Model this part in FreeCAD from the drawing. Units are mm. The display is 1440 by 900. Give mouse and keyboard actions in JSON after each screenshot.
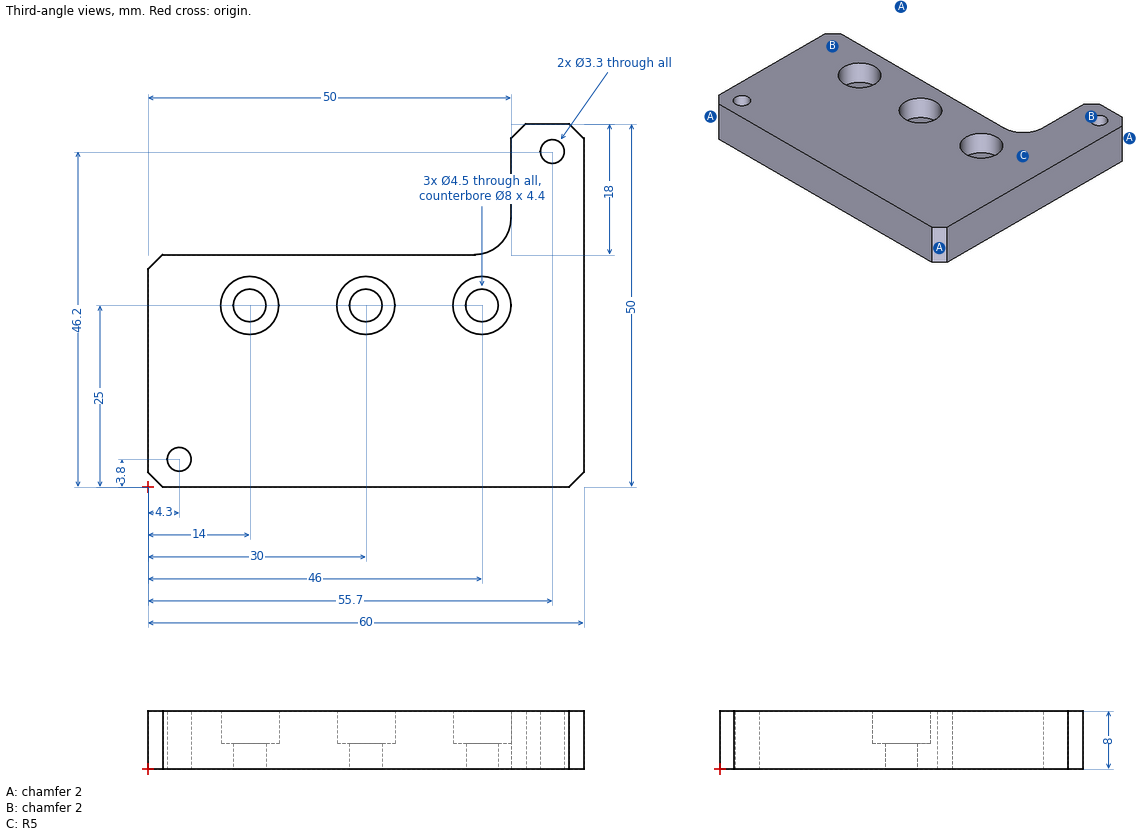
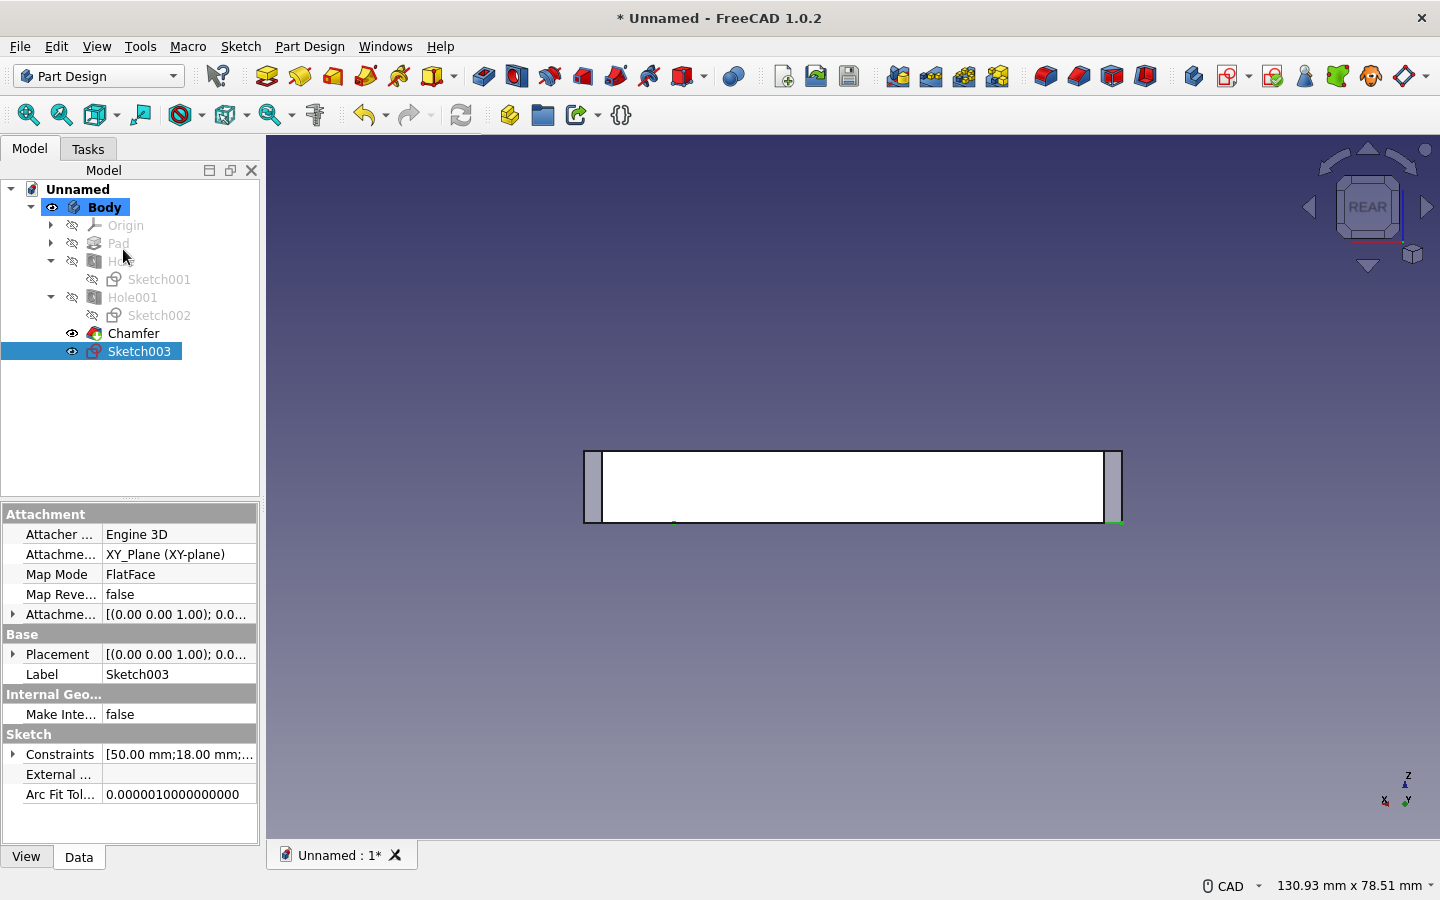
{"action": "left_click", "coordinate": [484, 76]}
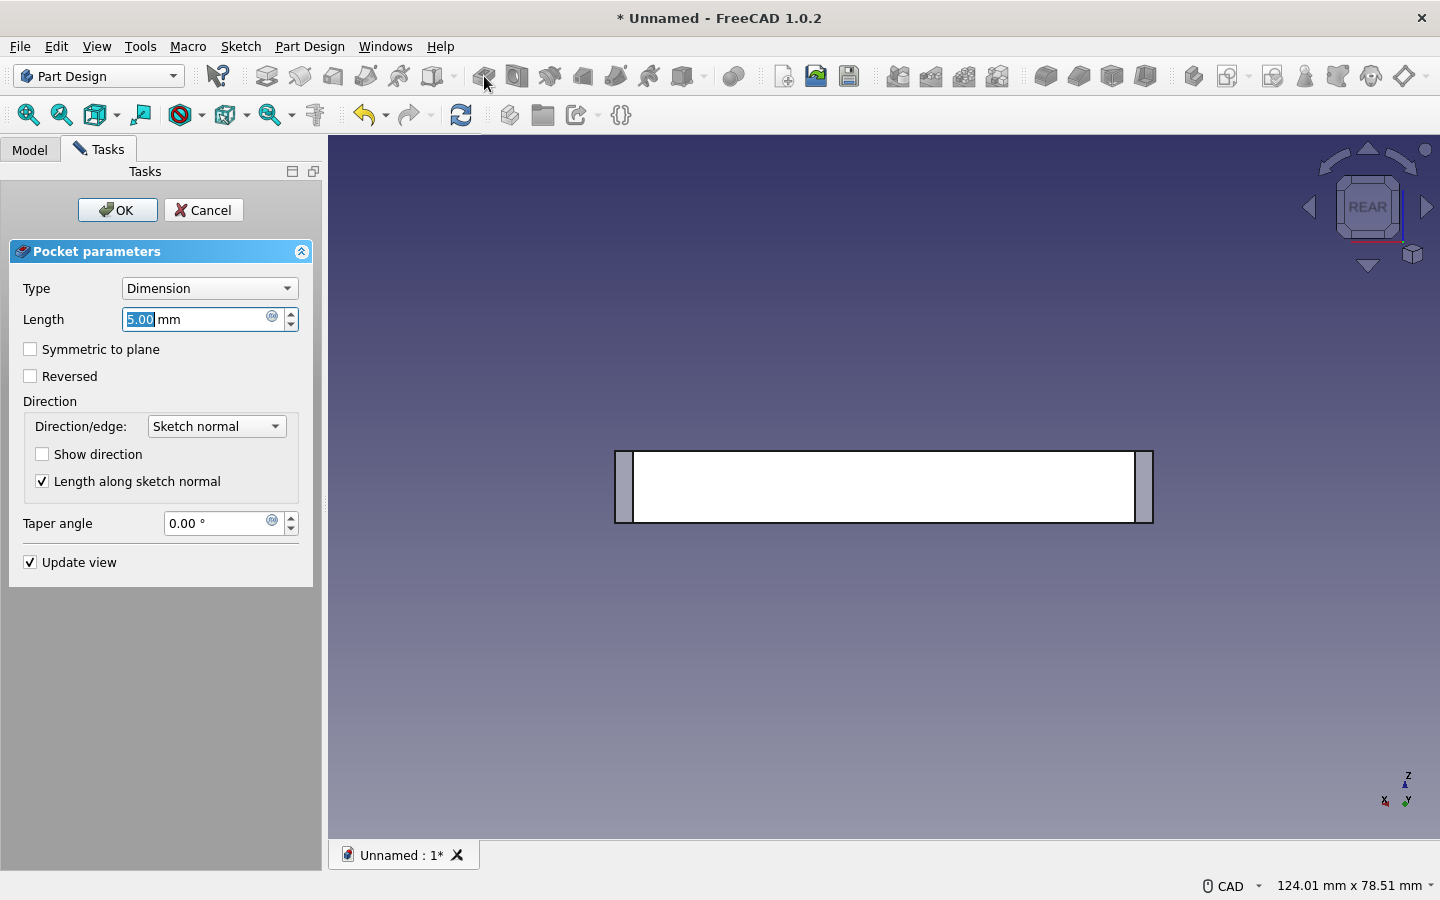
{"action": "left_click", "coordinate": [210, 288]}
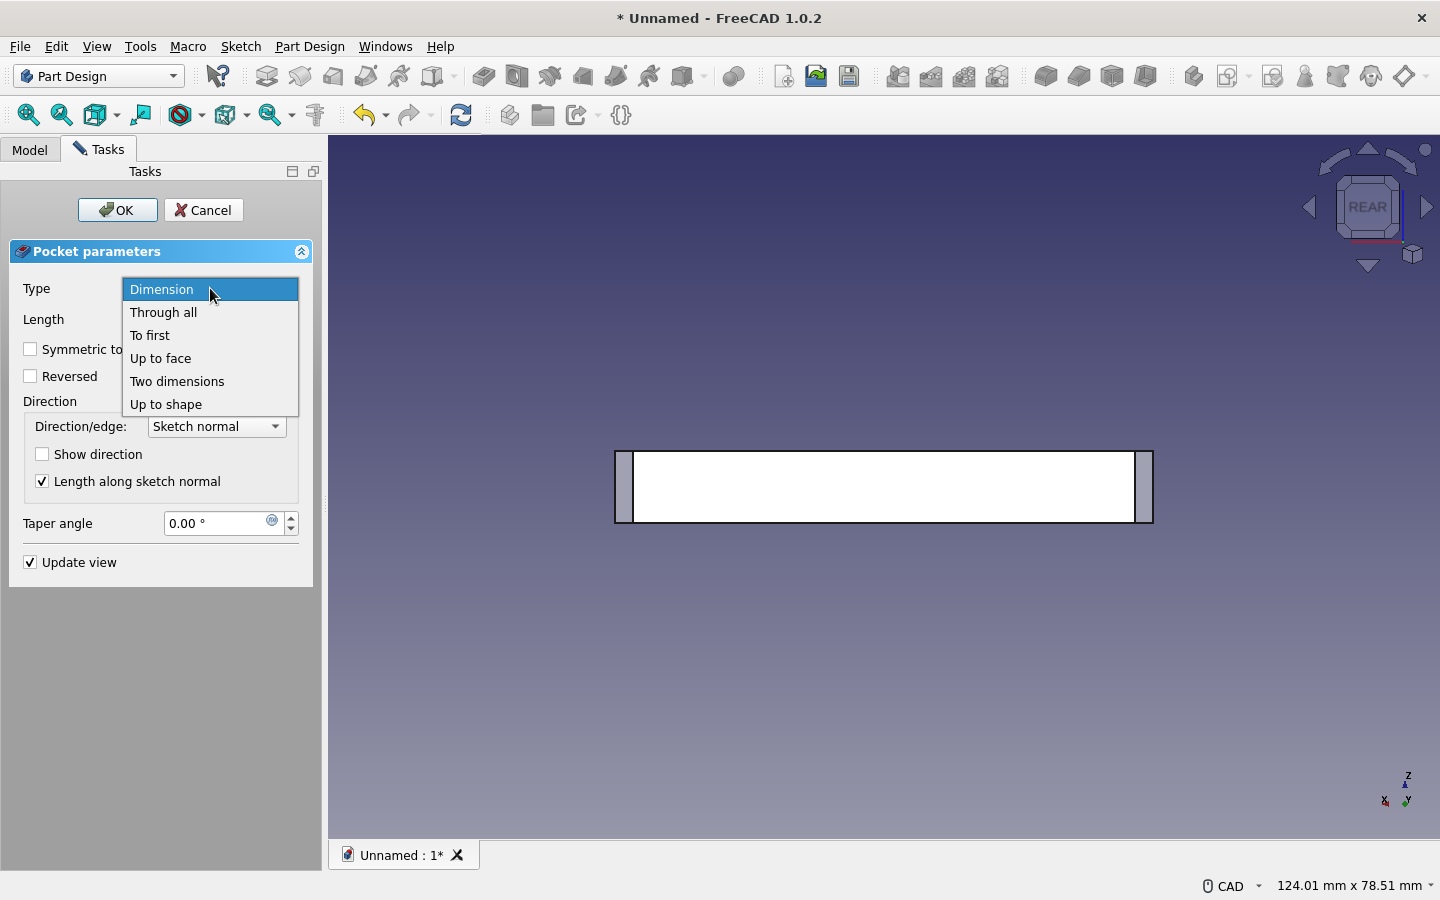
{"action": "left_click", "coordinate": [208, 312]}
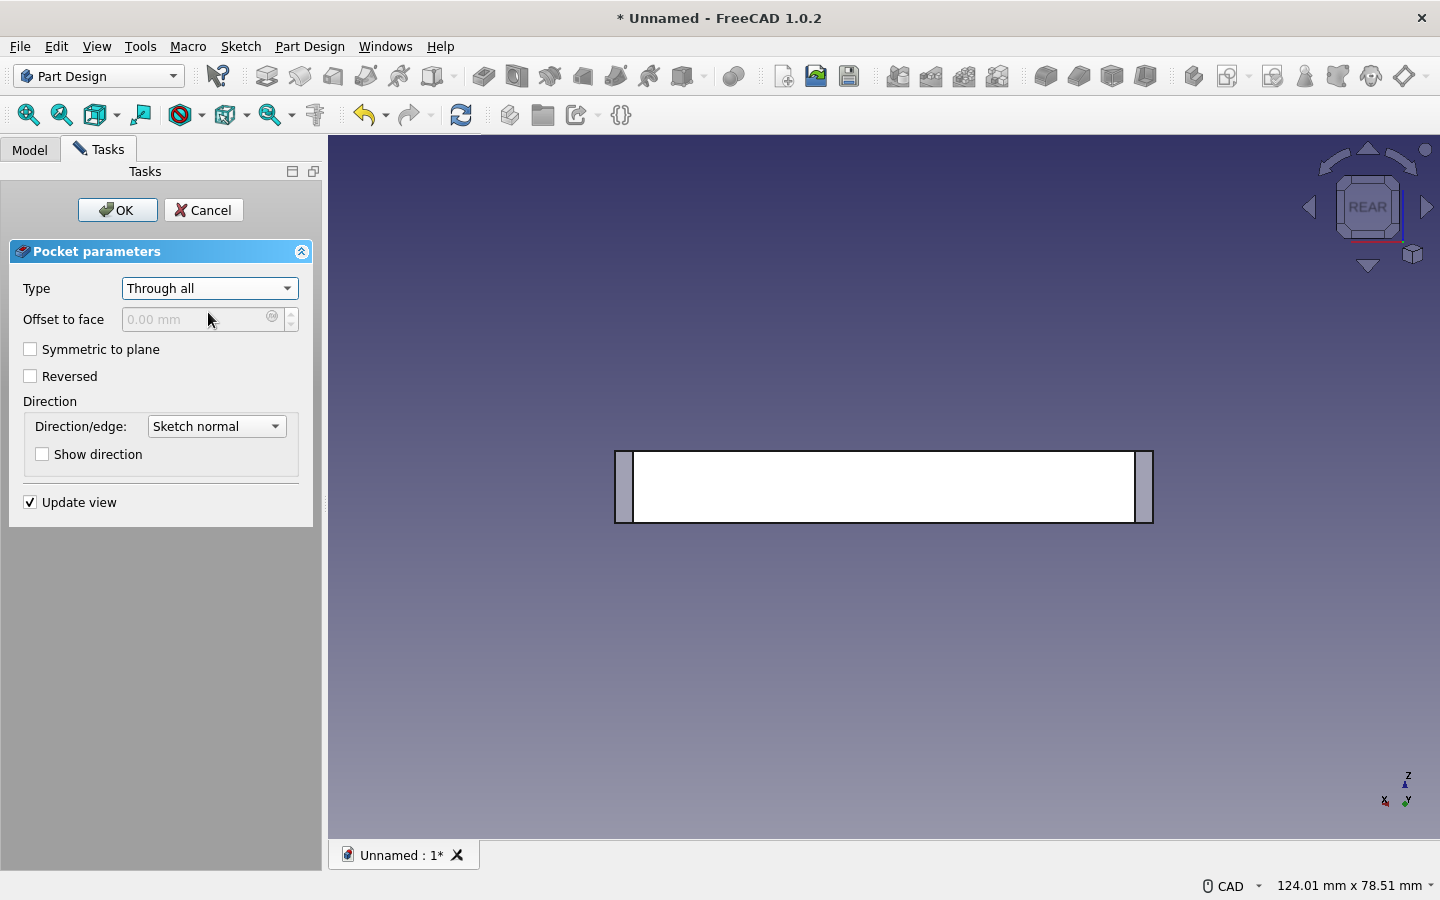
{"action": "left_click", "coordinate": [31, 376]}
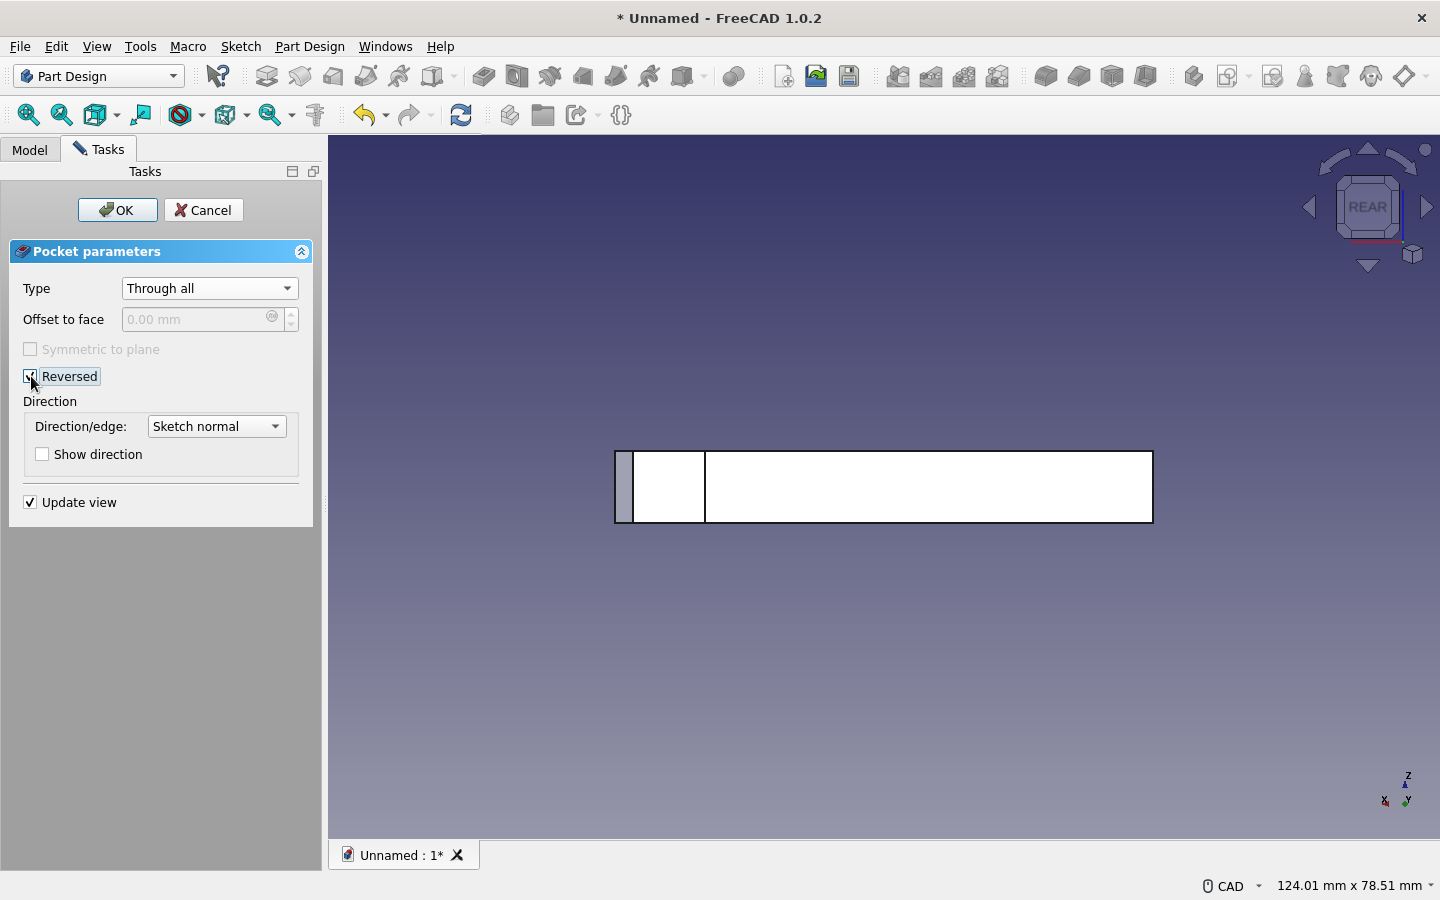
{"action": "left_click", "coordinate": [118, 210]}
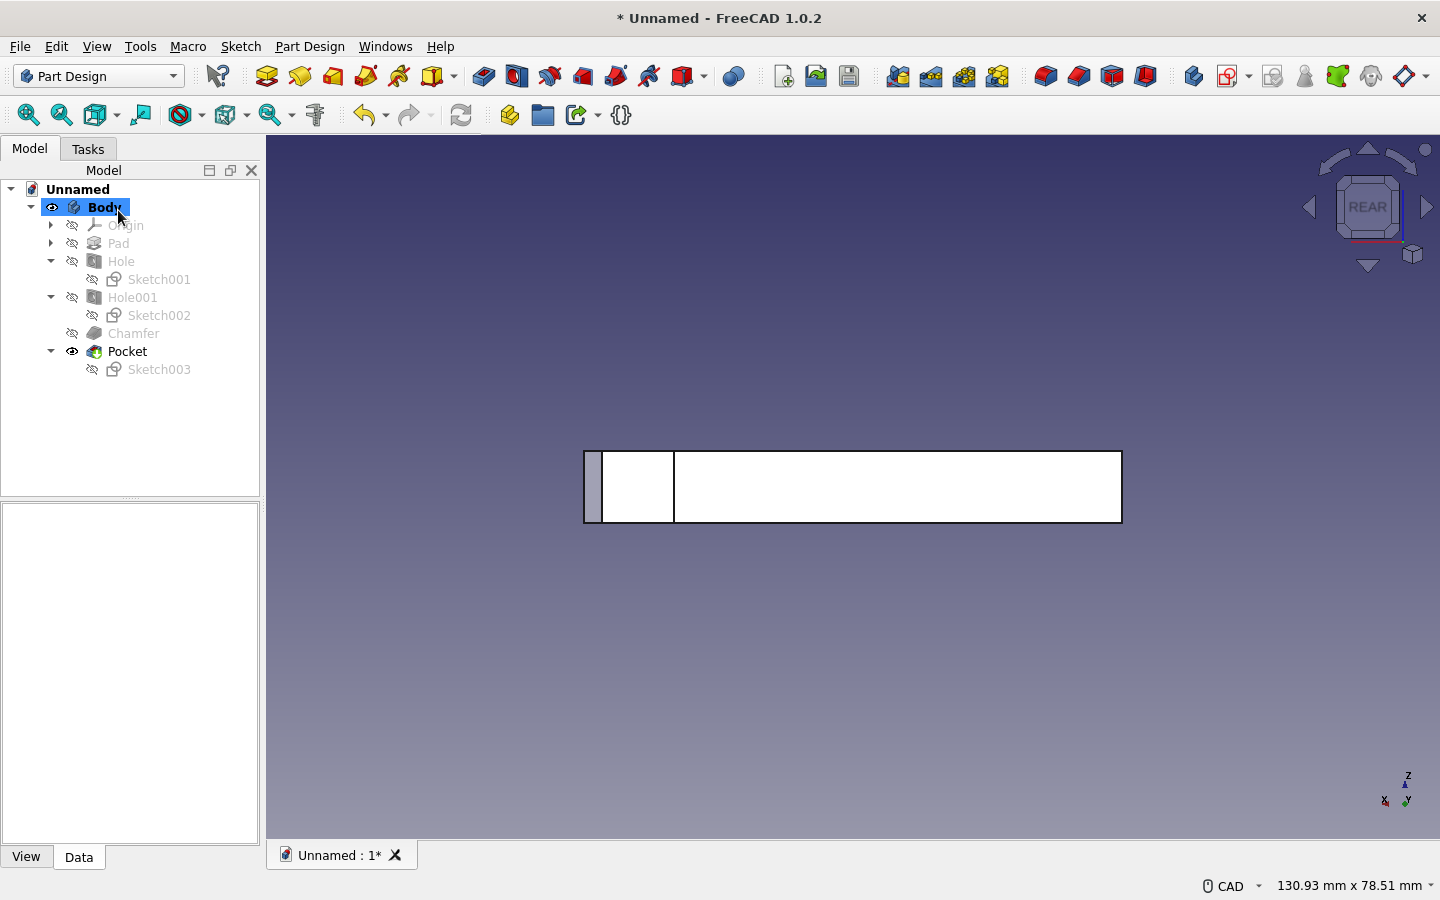
{"action": "left_click", "coordinate": [674, 486]}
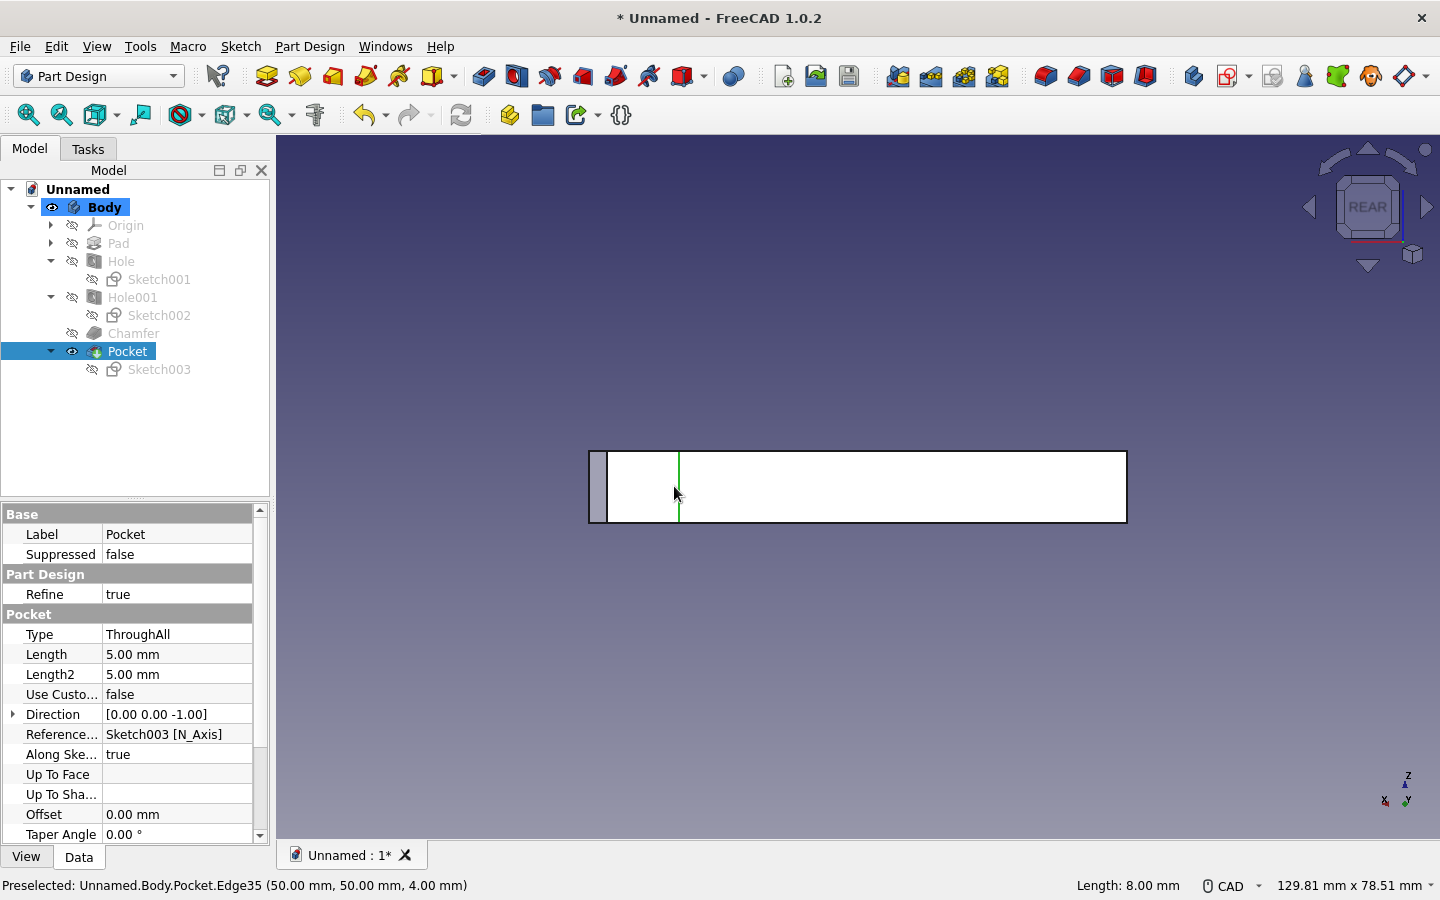
{"action": "left_click", "coordinate": [1127, 486], "text": "ctrl"}